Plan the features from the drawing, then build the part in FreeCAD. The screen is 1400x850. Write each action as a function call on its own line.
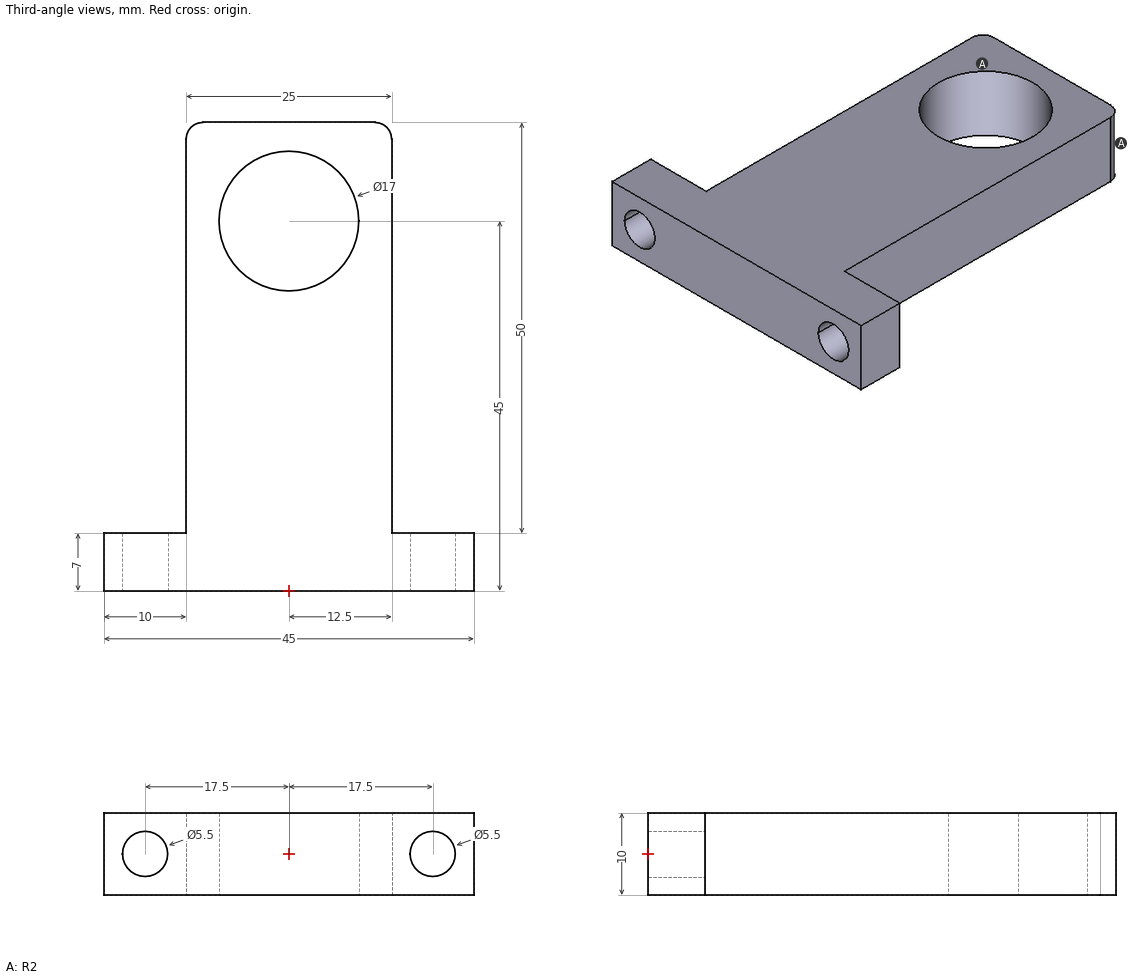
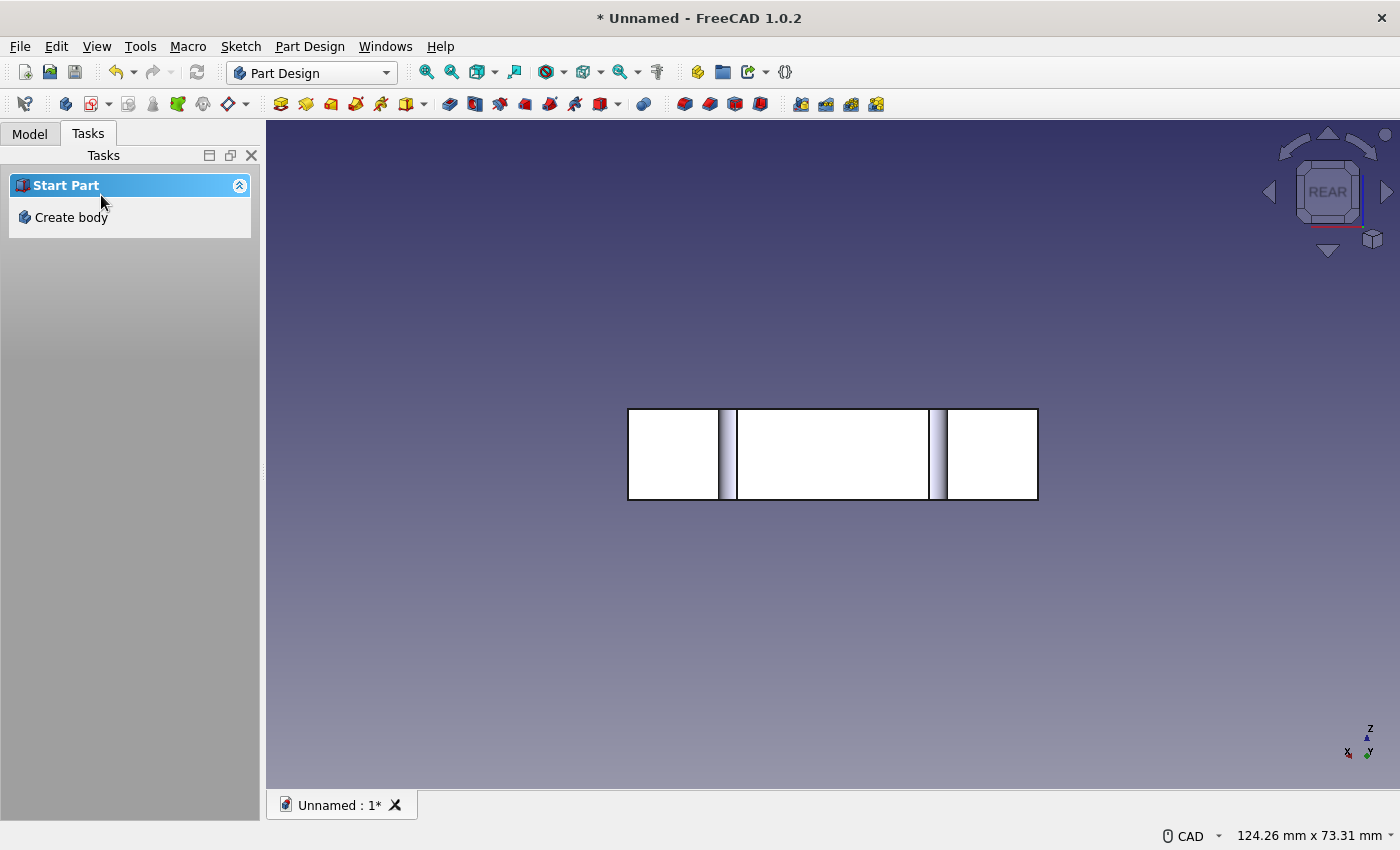
key(v)
key(f)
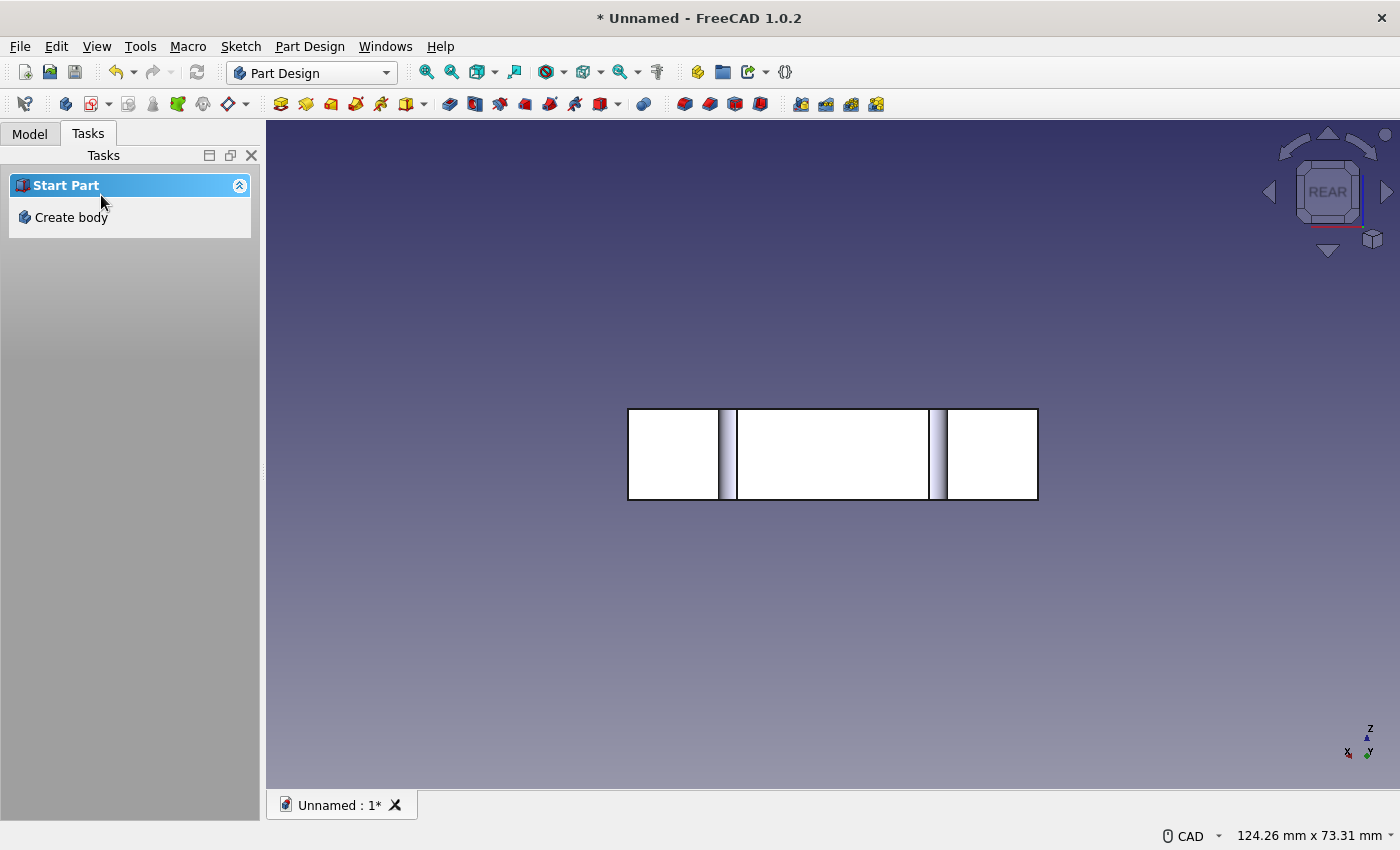
click(673, 454)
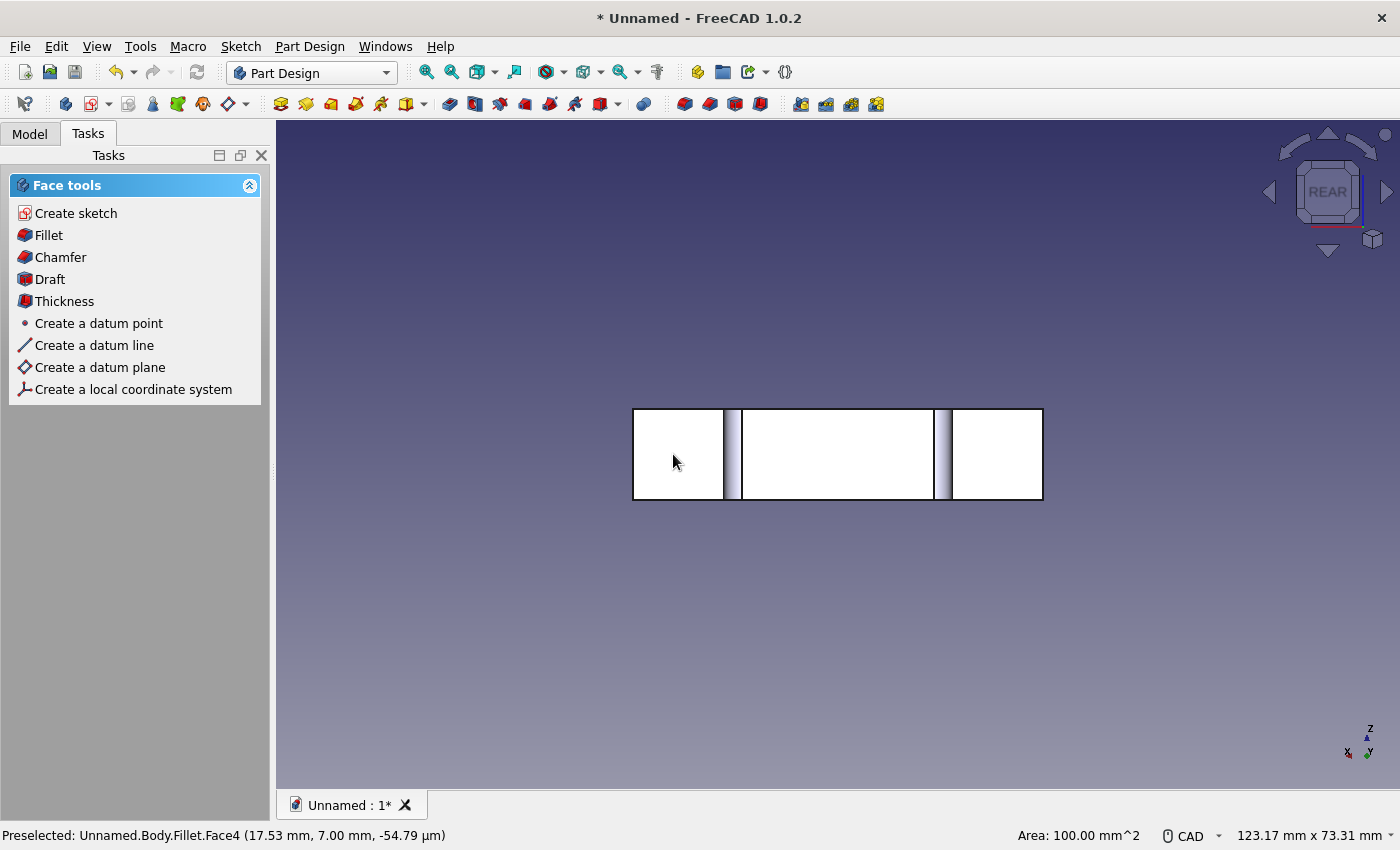
click(90, 104)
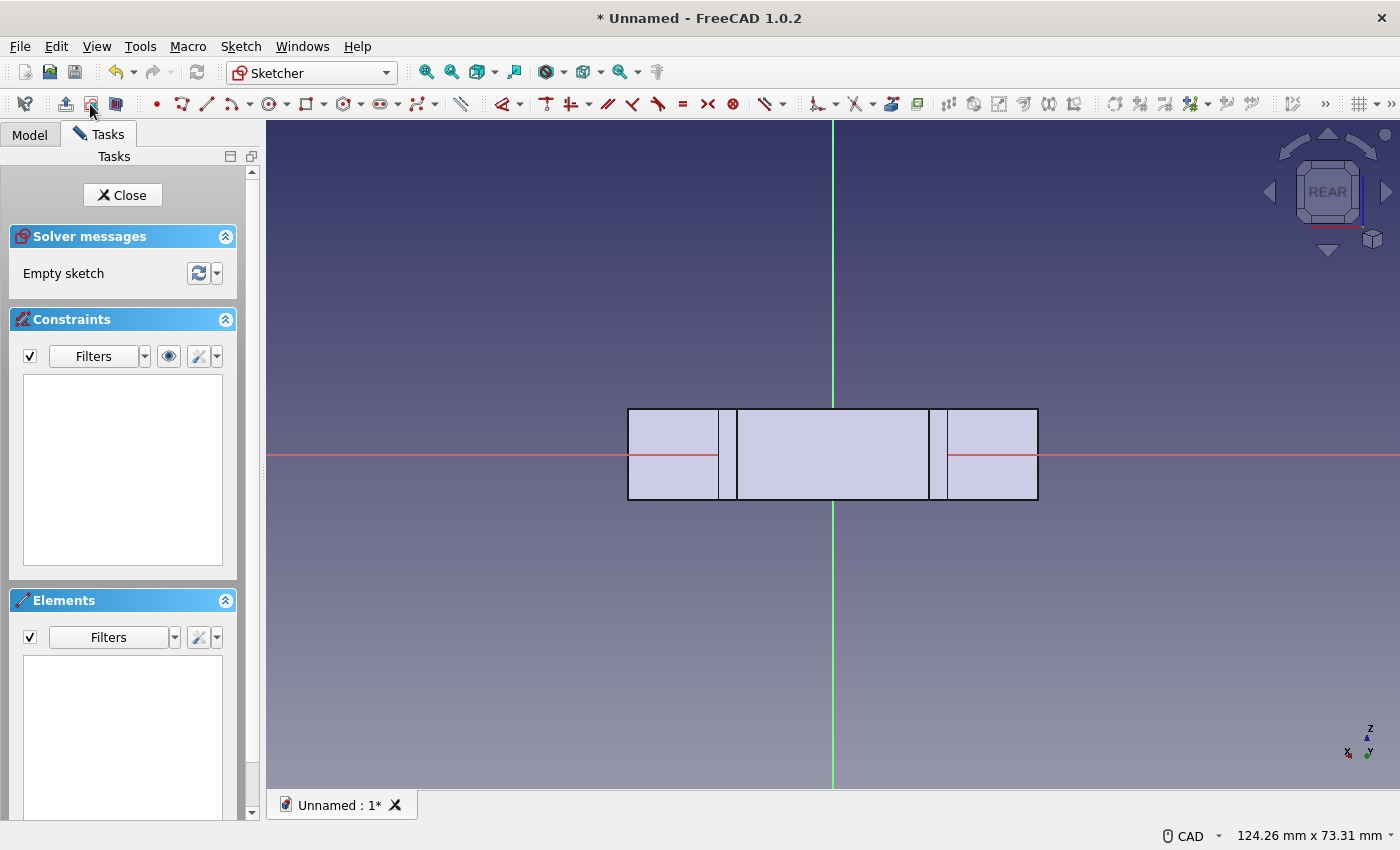
key(q)
key(s)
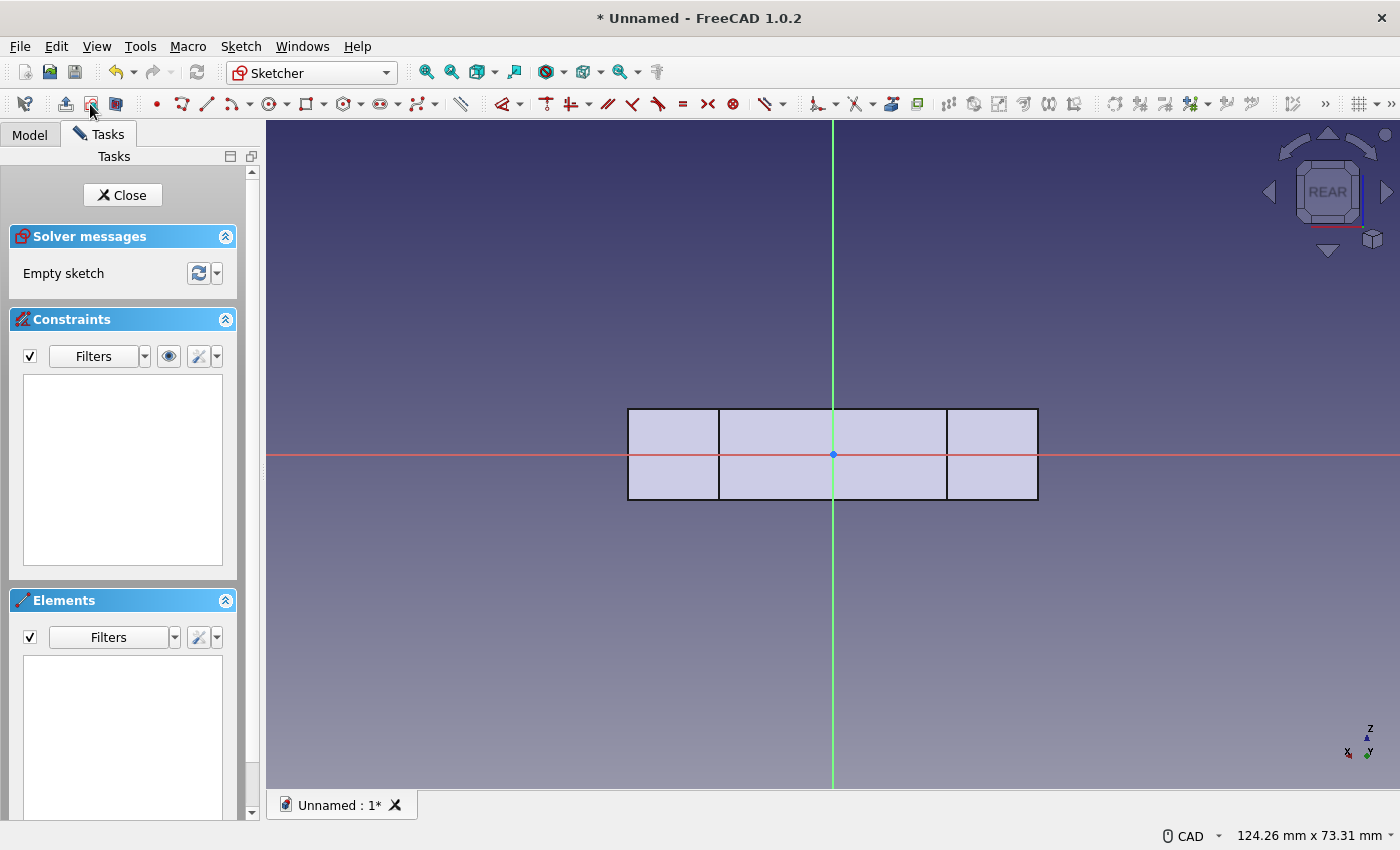
scroll(1021, 454, up, 11)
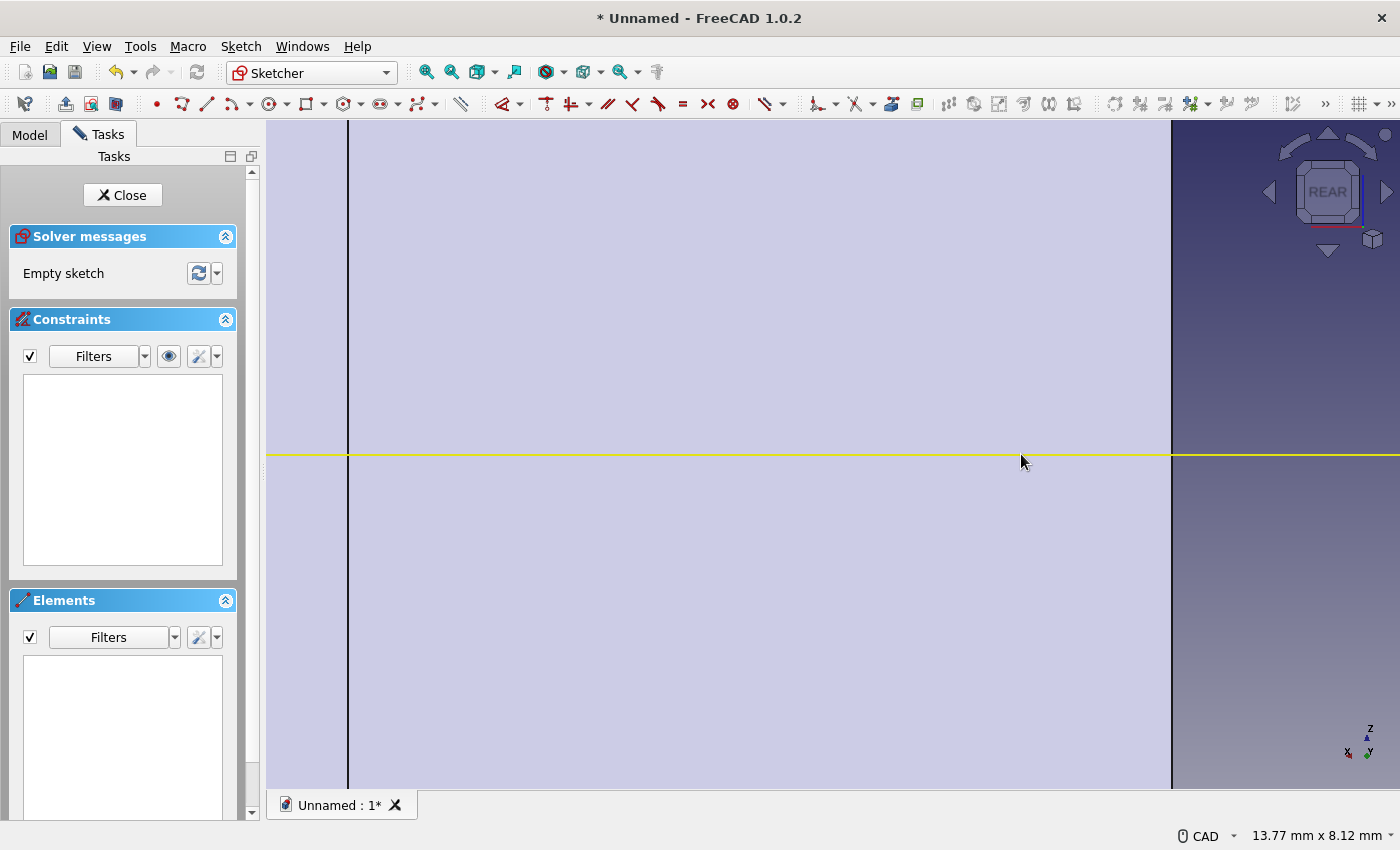
key(g)
key(c)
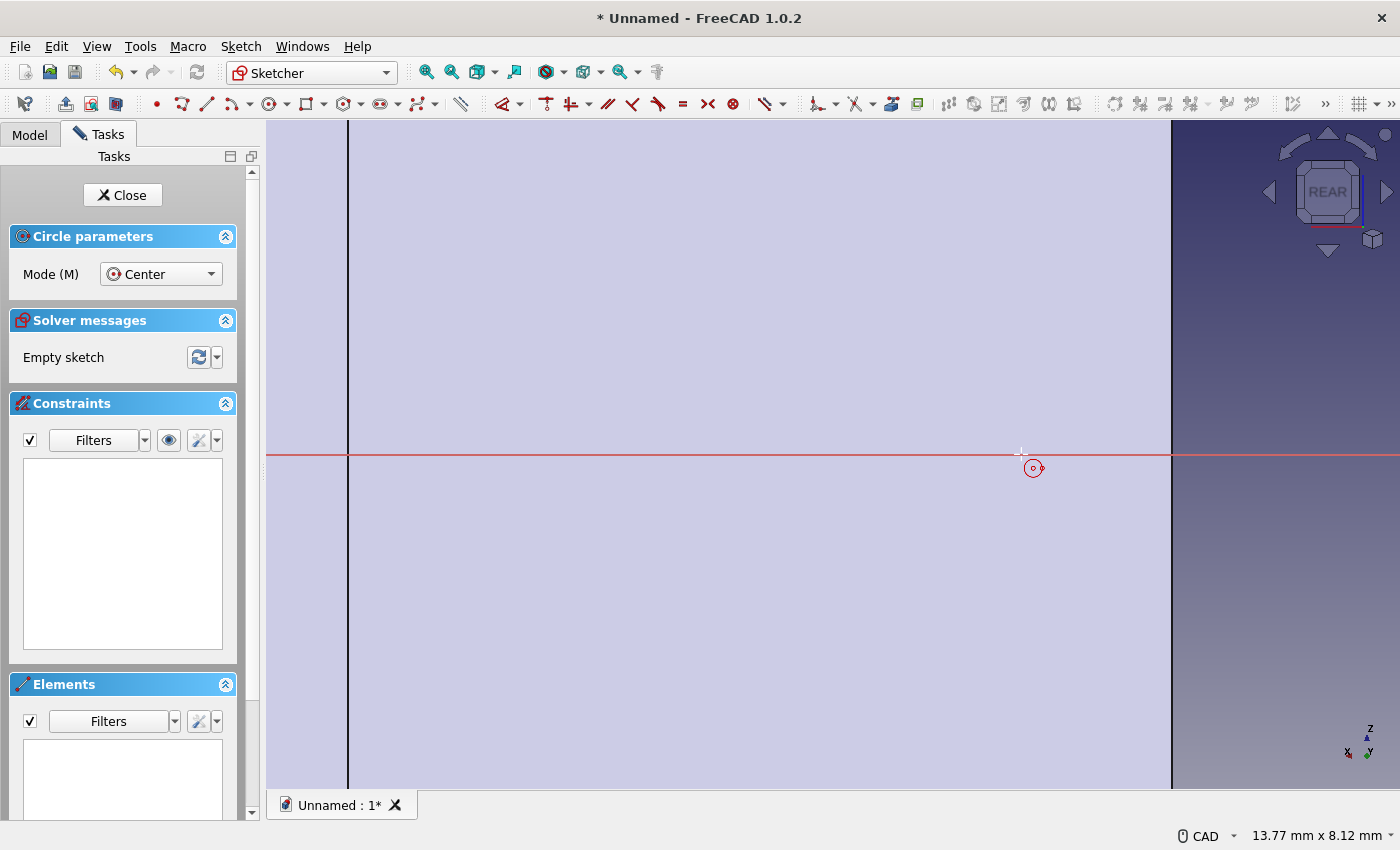
click(760, 454)
click(920, 294)
key(Escape)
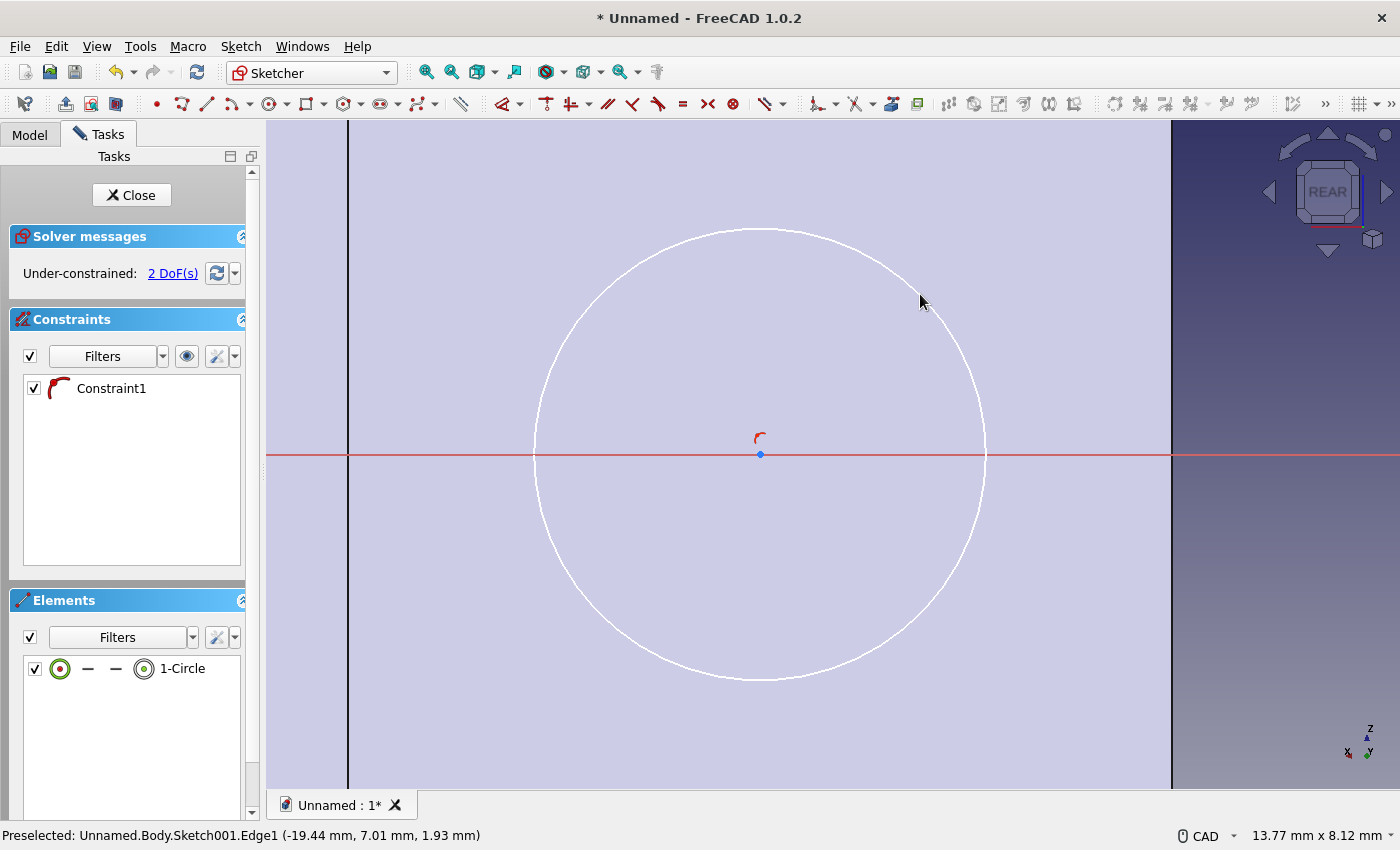
click(502, 104)